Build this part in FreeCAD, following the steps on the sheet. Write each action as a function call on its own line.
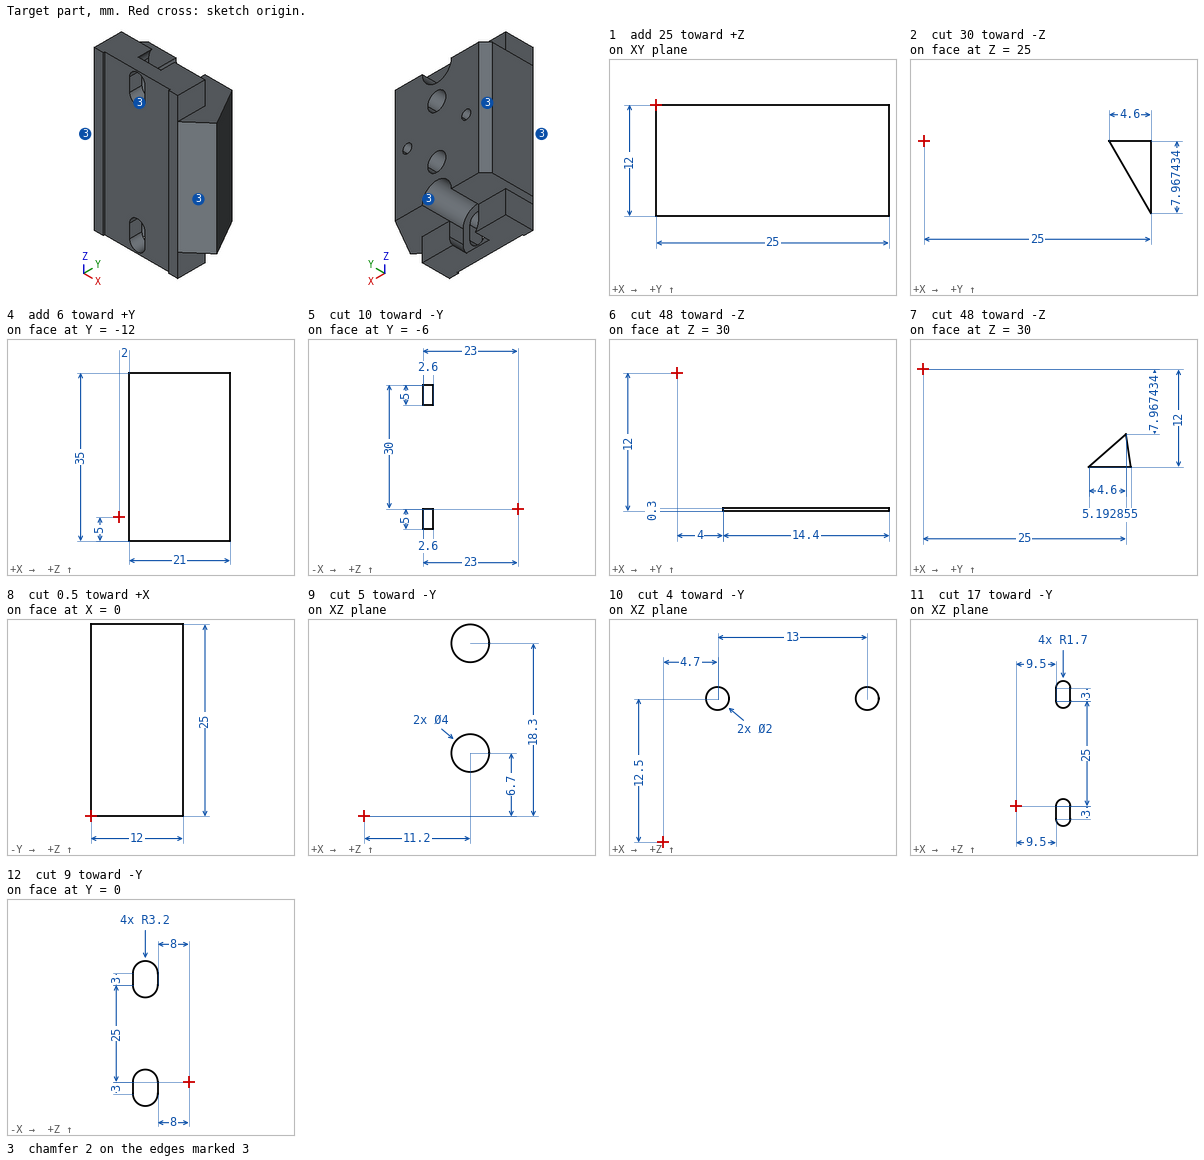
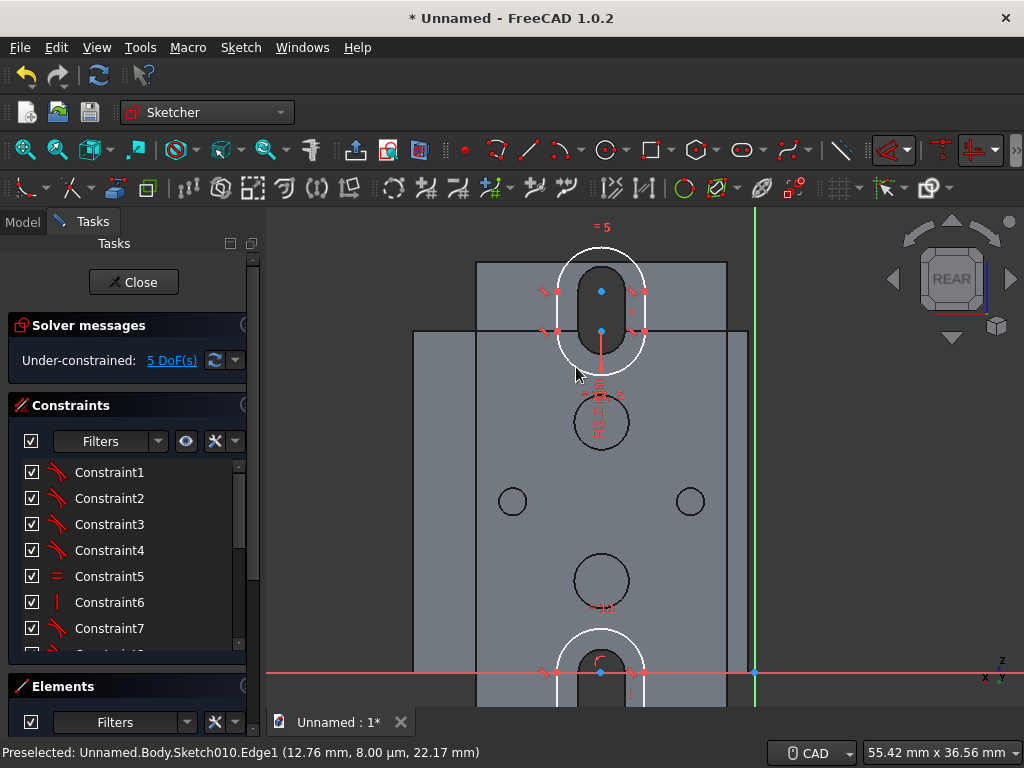
click(557, 319)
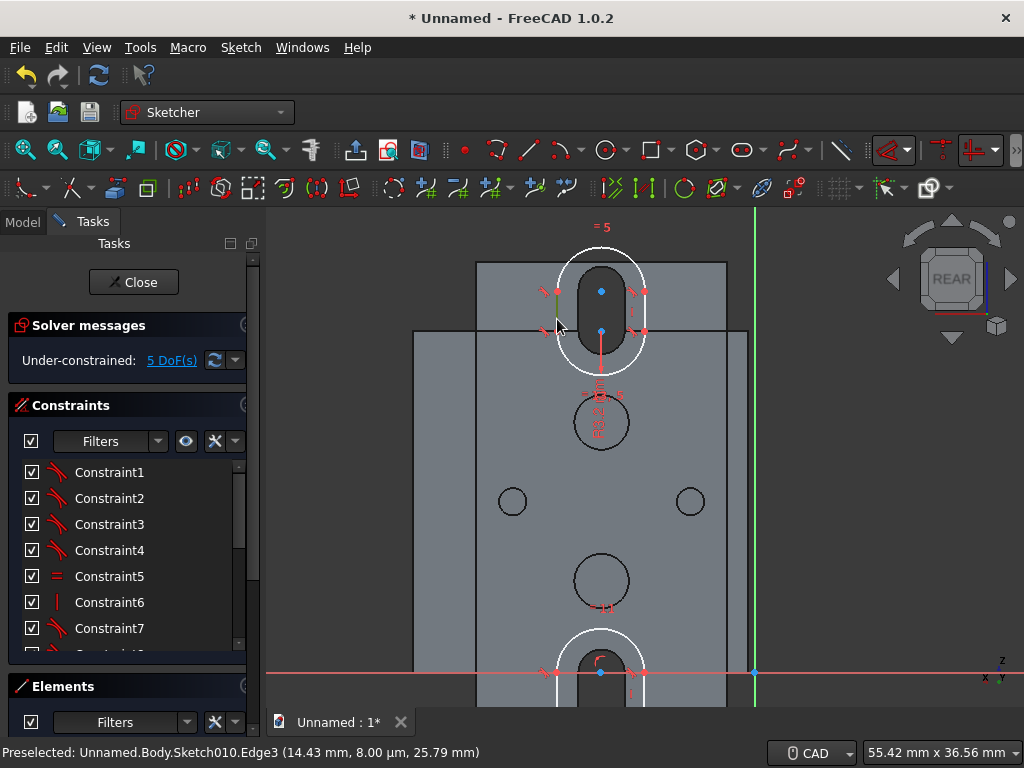
click(910, 150)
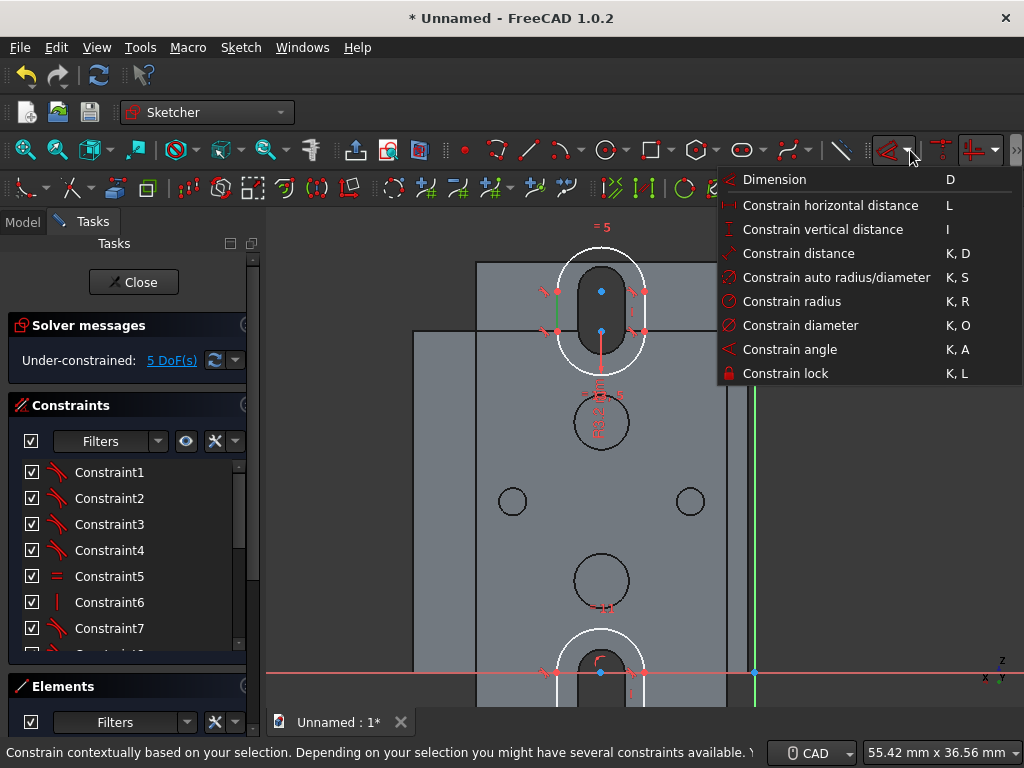
click(870, 229)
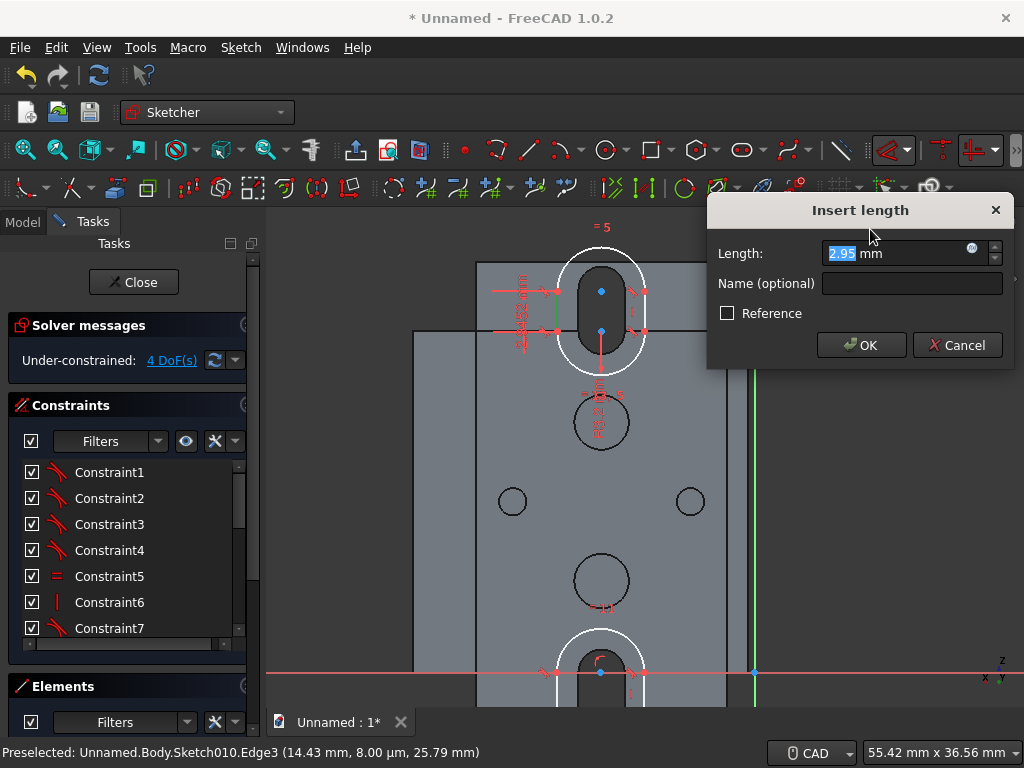
text(3)
key(Return)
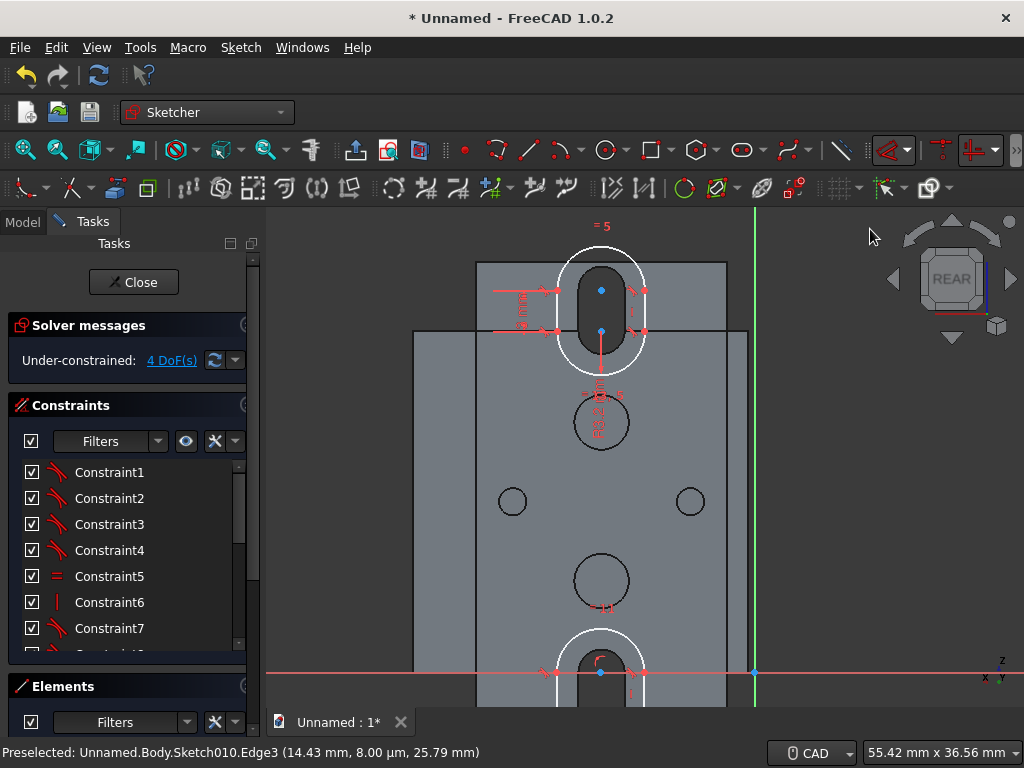
scroll(414, 366, down, 2)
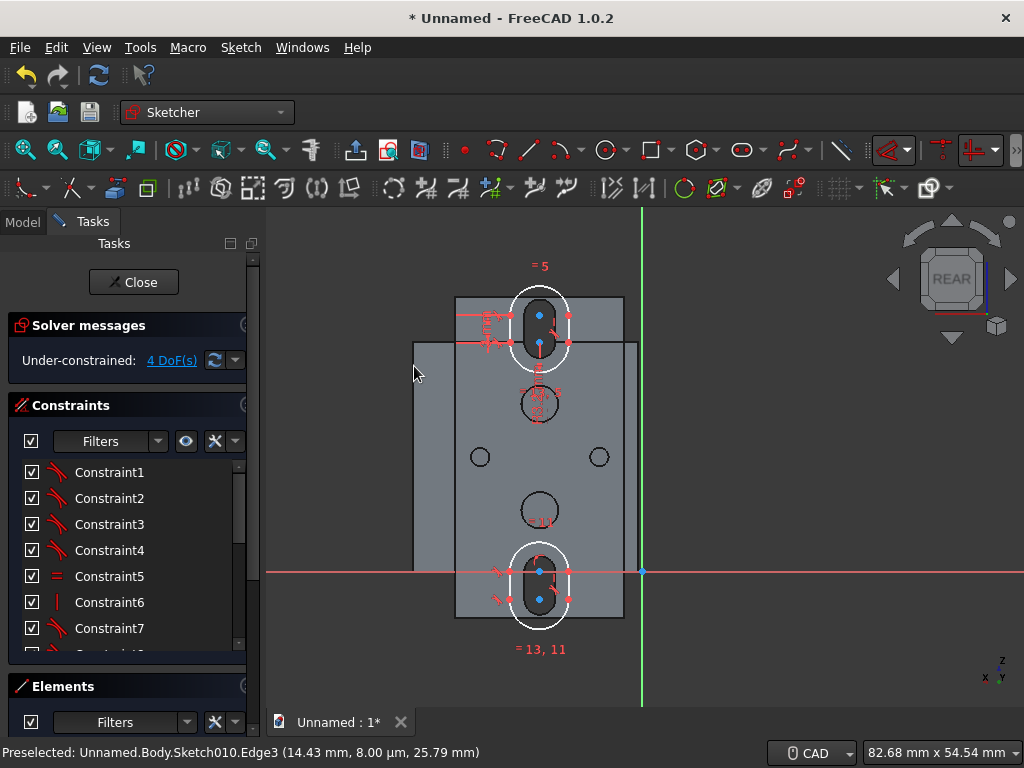
scroll(510, 592, up, 3)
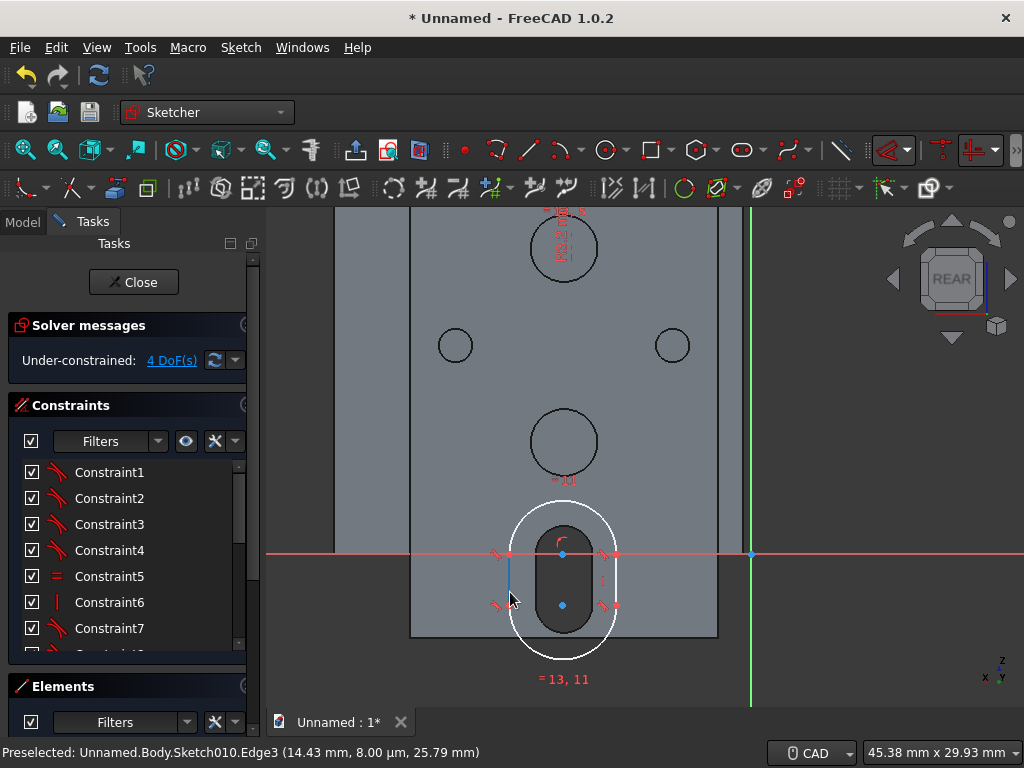
click(509, 590)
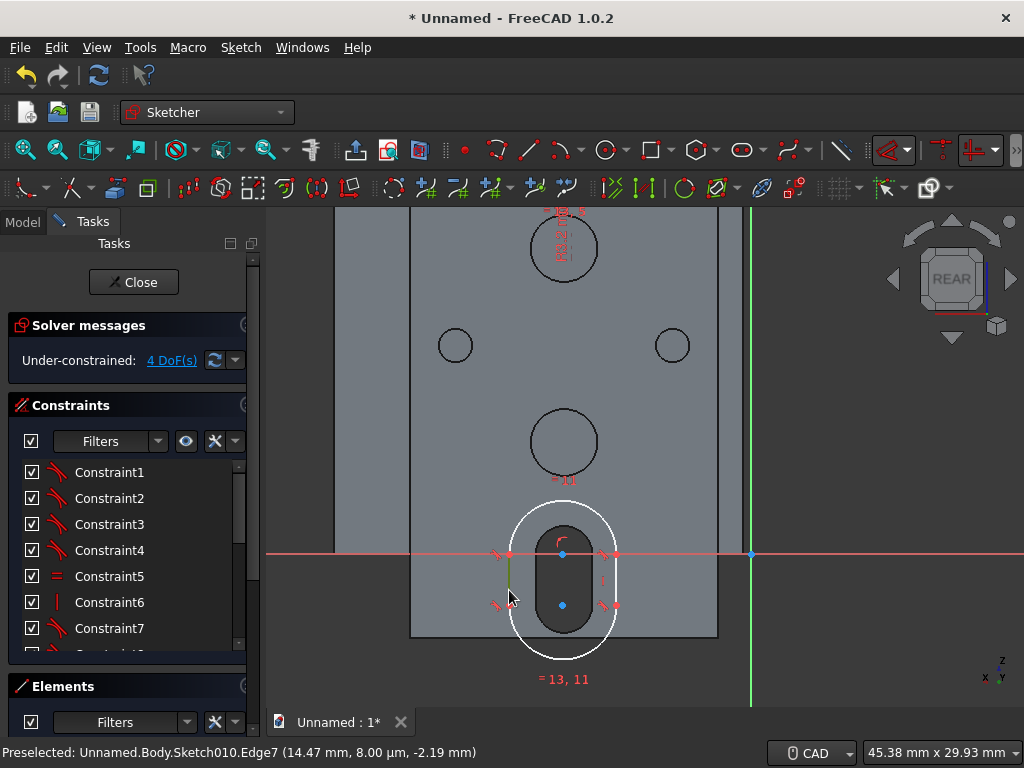
click(910, 150)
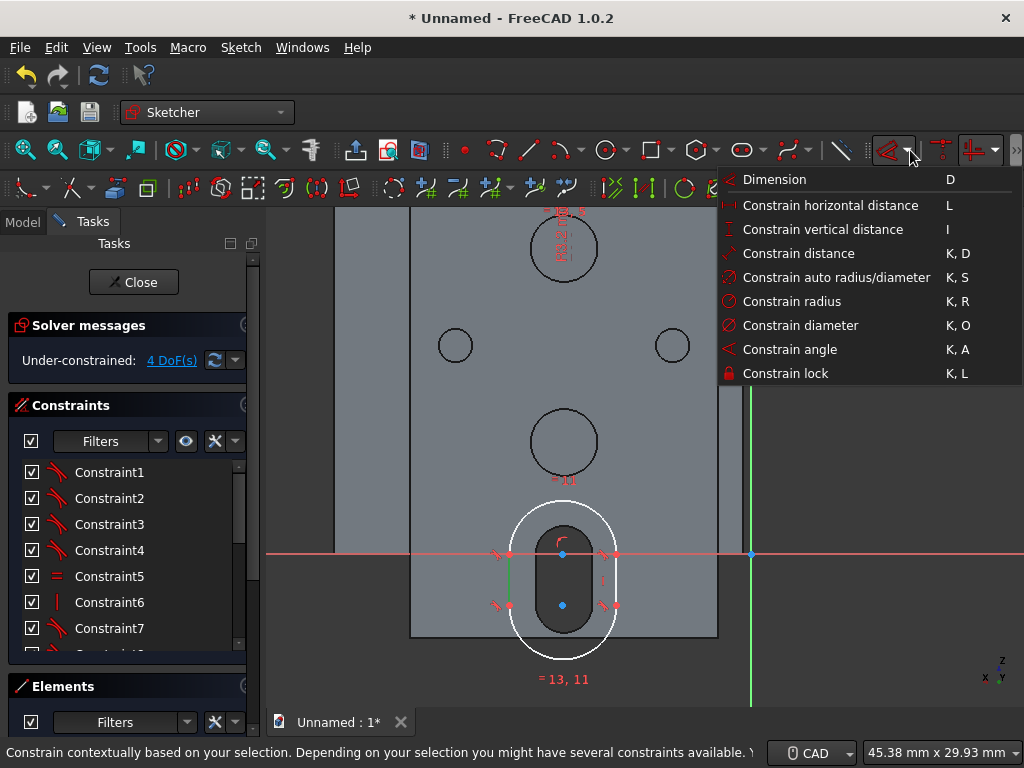
click(870, 229)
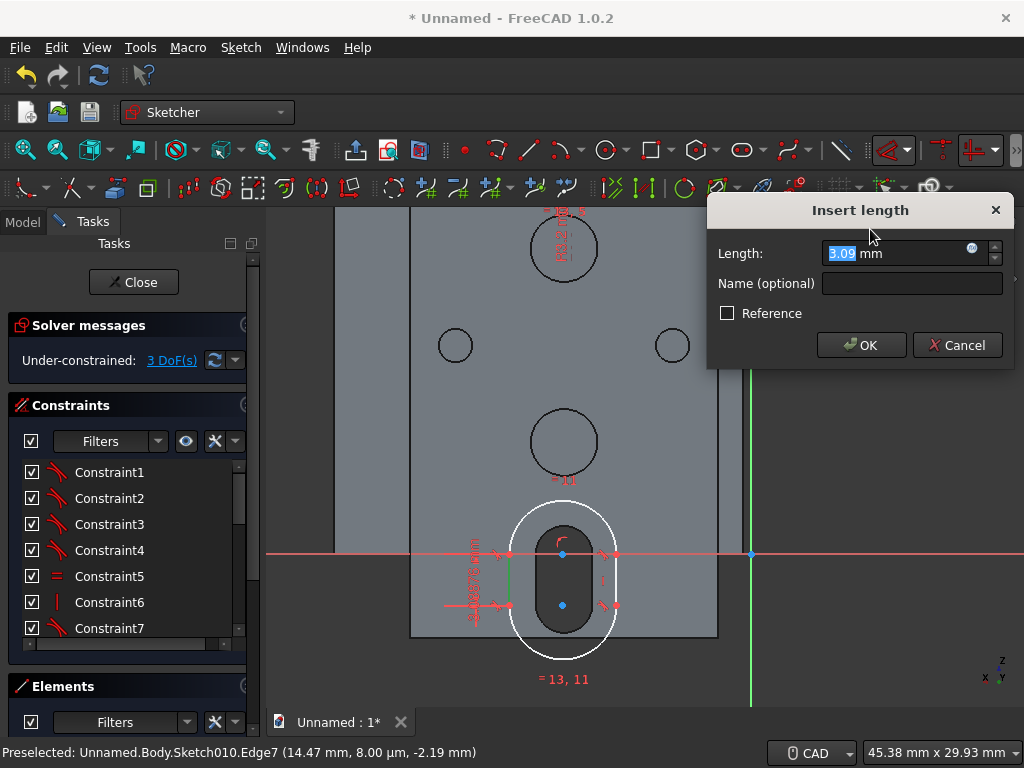
text(3)
key(Return)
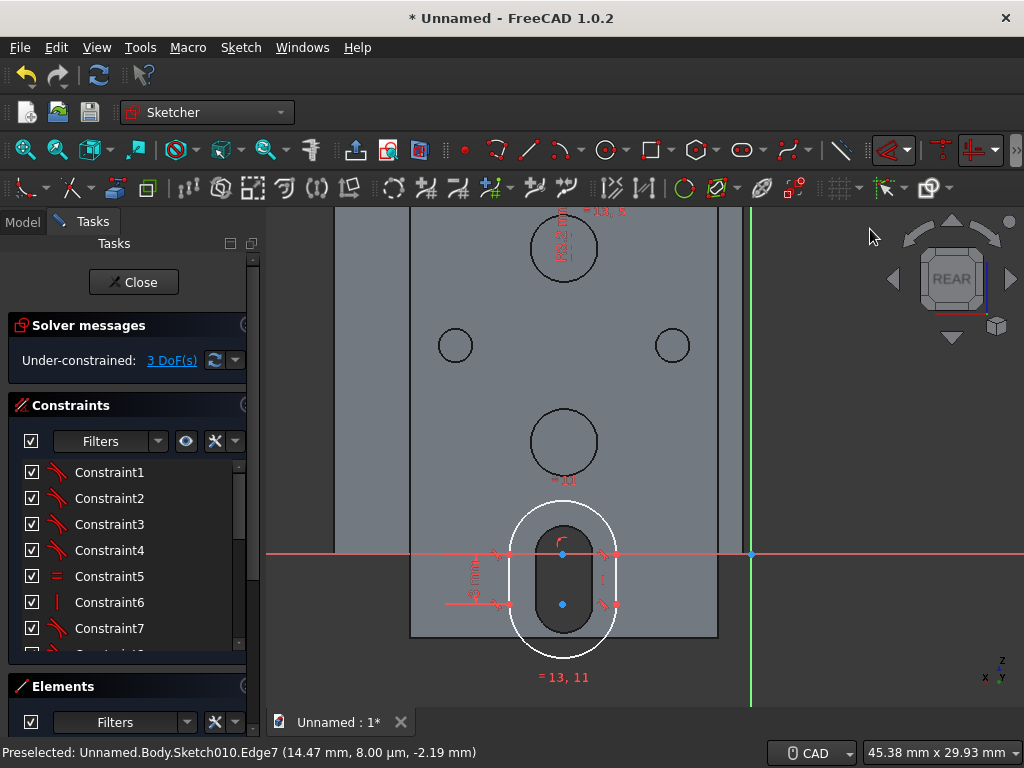
scroll(510, 593, down, 3)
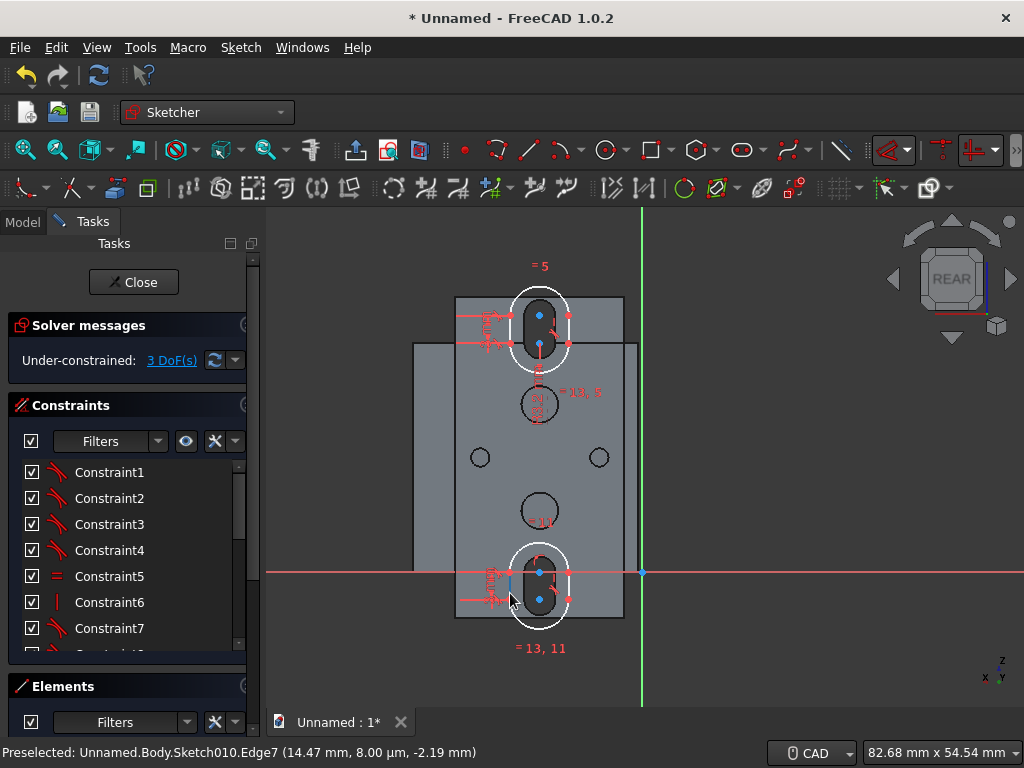
click(569, 343)